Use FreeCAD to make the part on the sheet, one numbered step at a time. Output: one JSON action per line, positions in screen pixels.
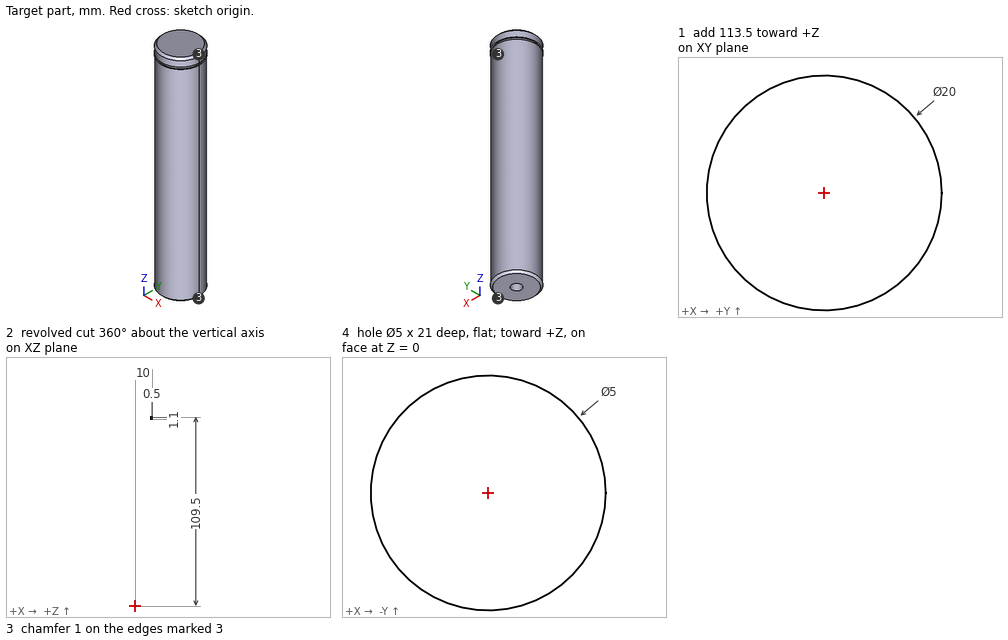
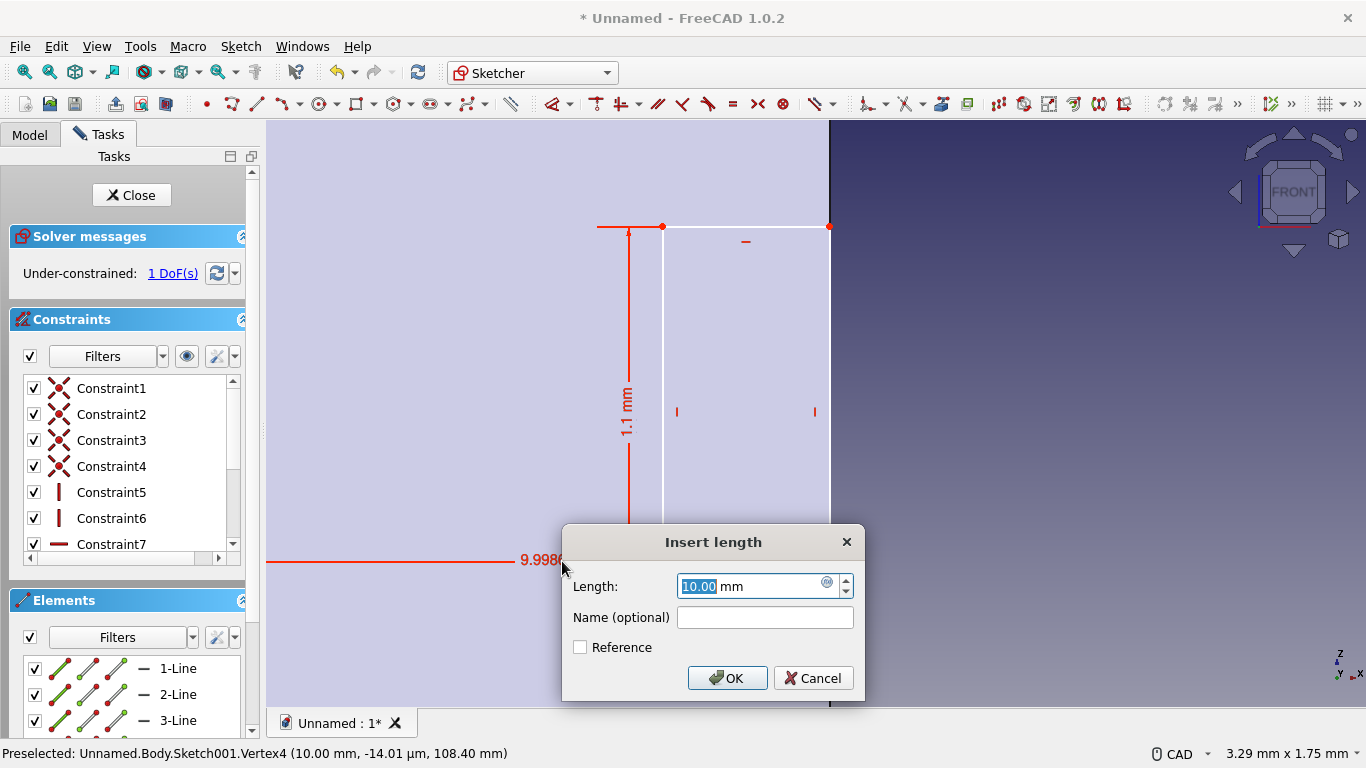
{"action": "type", "text": "10"}
{"action": "key", "text": "Return"}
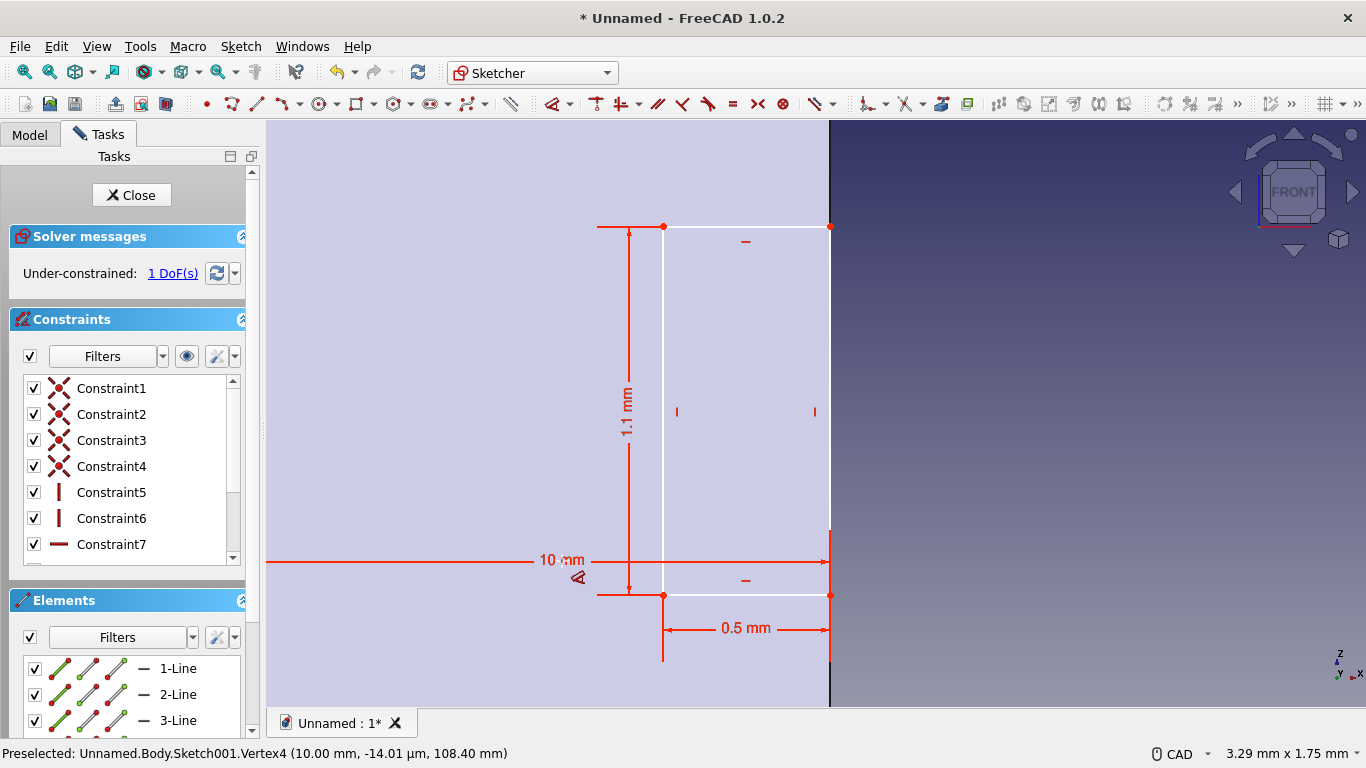
{"action": "left_click", "coordinate": [663, 227]}
{"action": "left_click", "coordinate": [697, 453]}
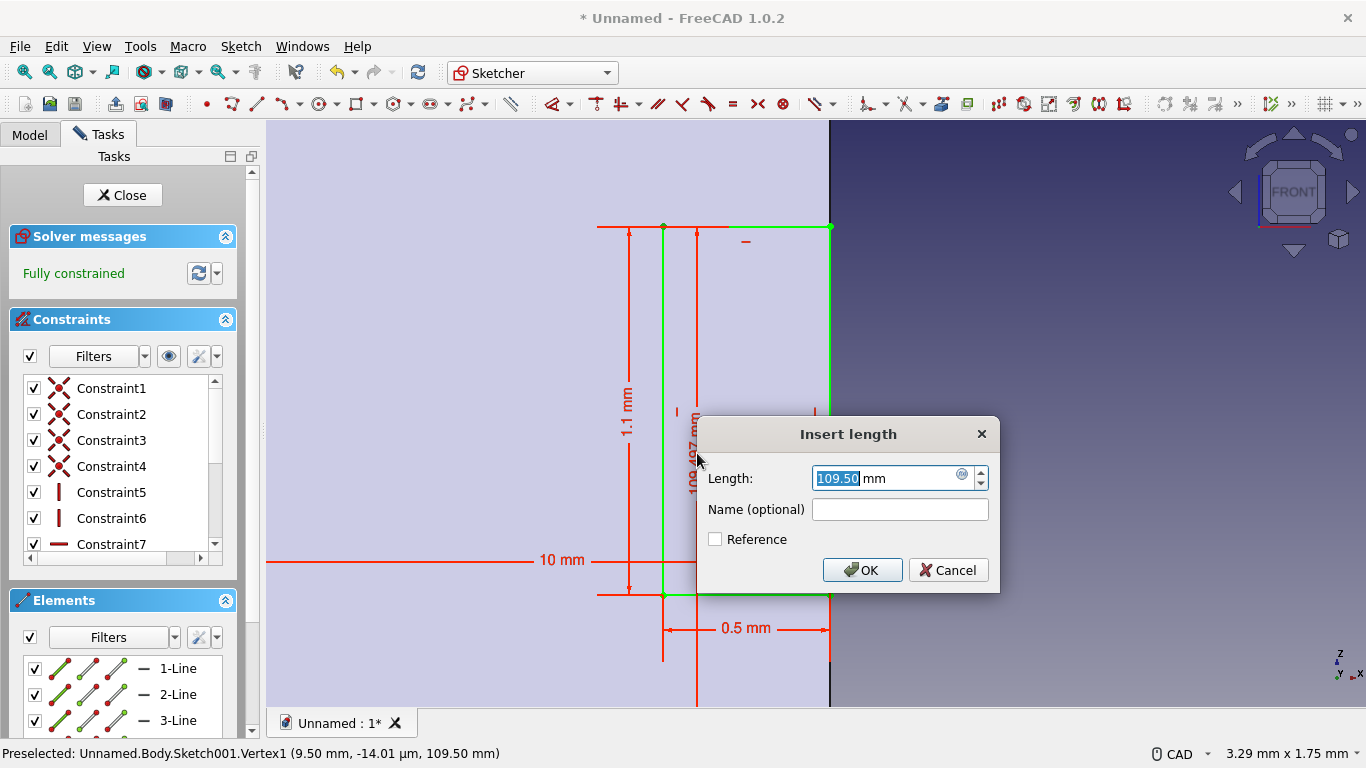
{"action": "type", "text": "109.5"}
{"action": "key", "text": "Return"}
{"action": "key", "text": "Escape"}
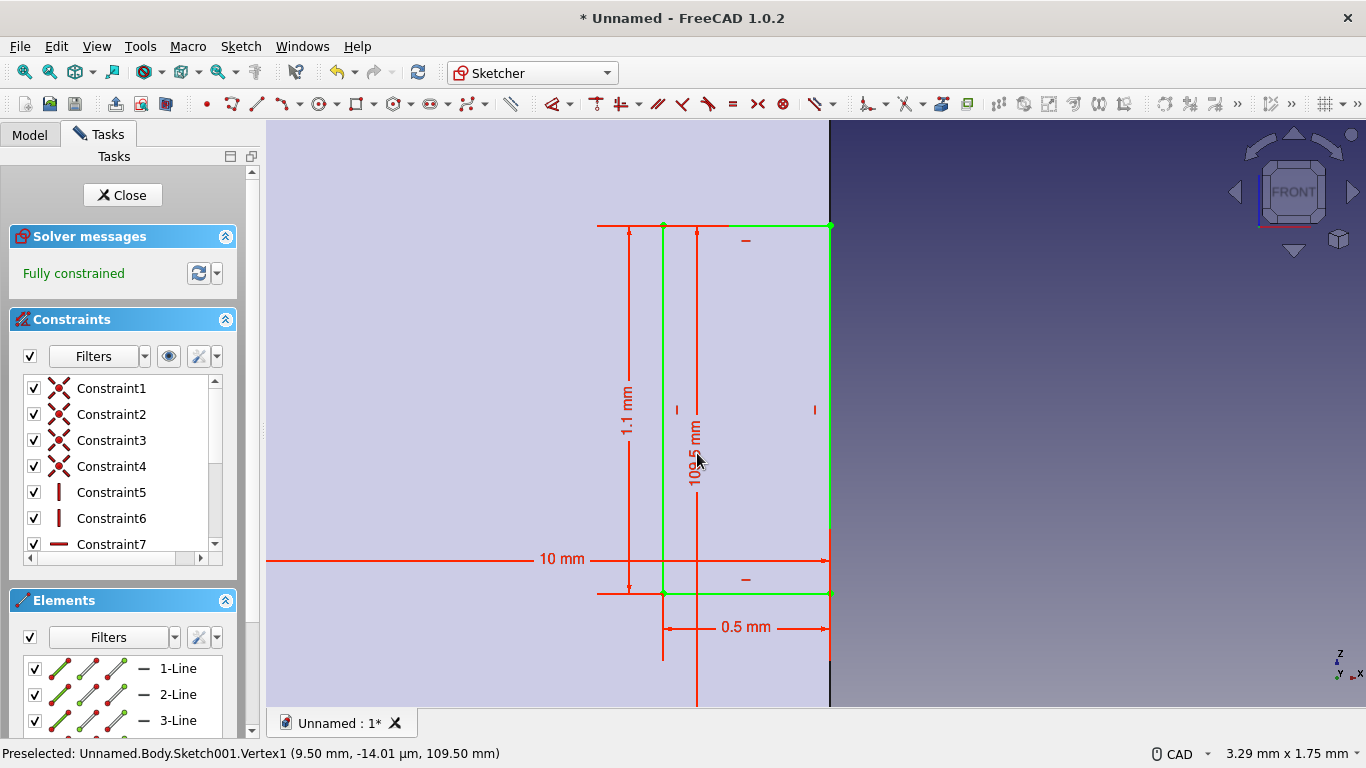
{"action": "left_click", "coordinate": [123, 195]}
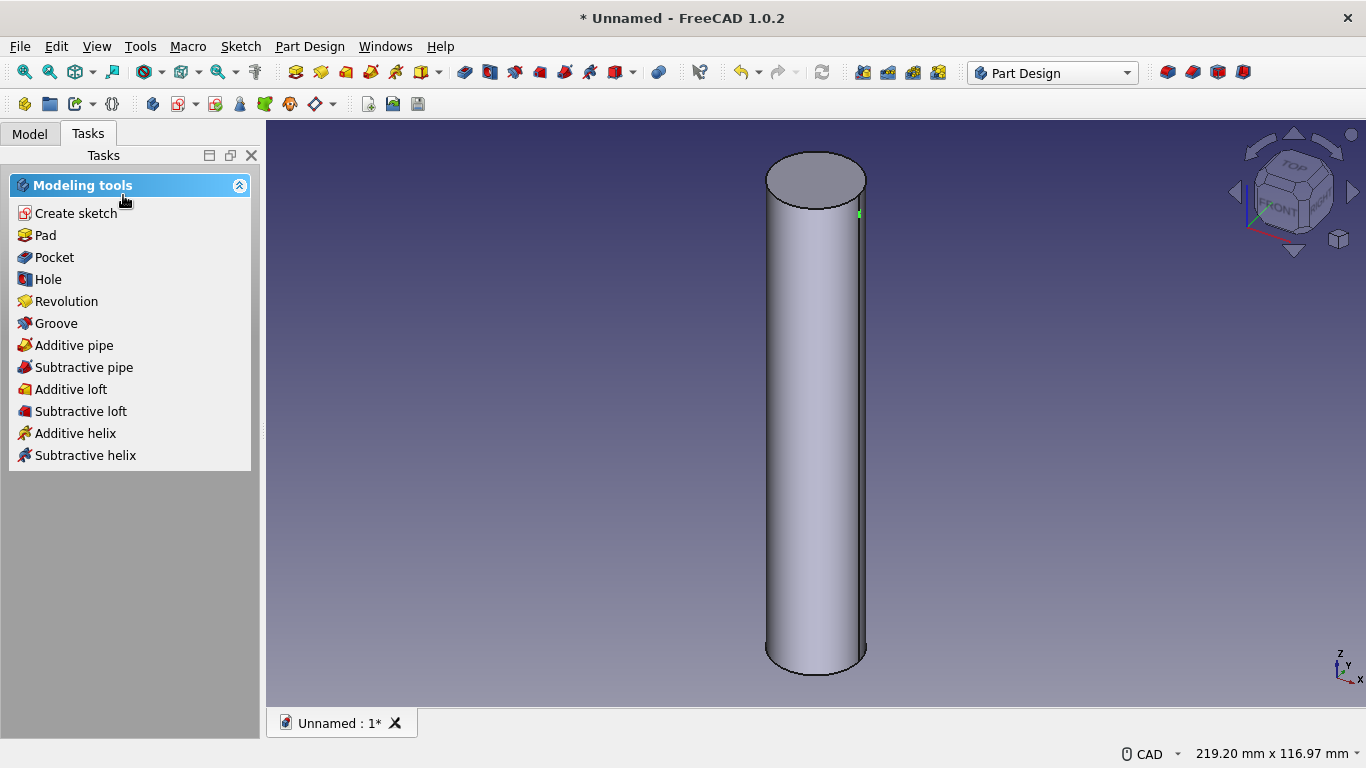
{"action": "left_click", "coordinate": [515, 72]}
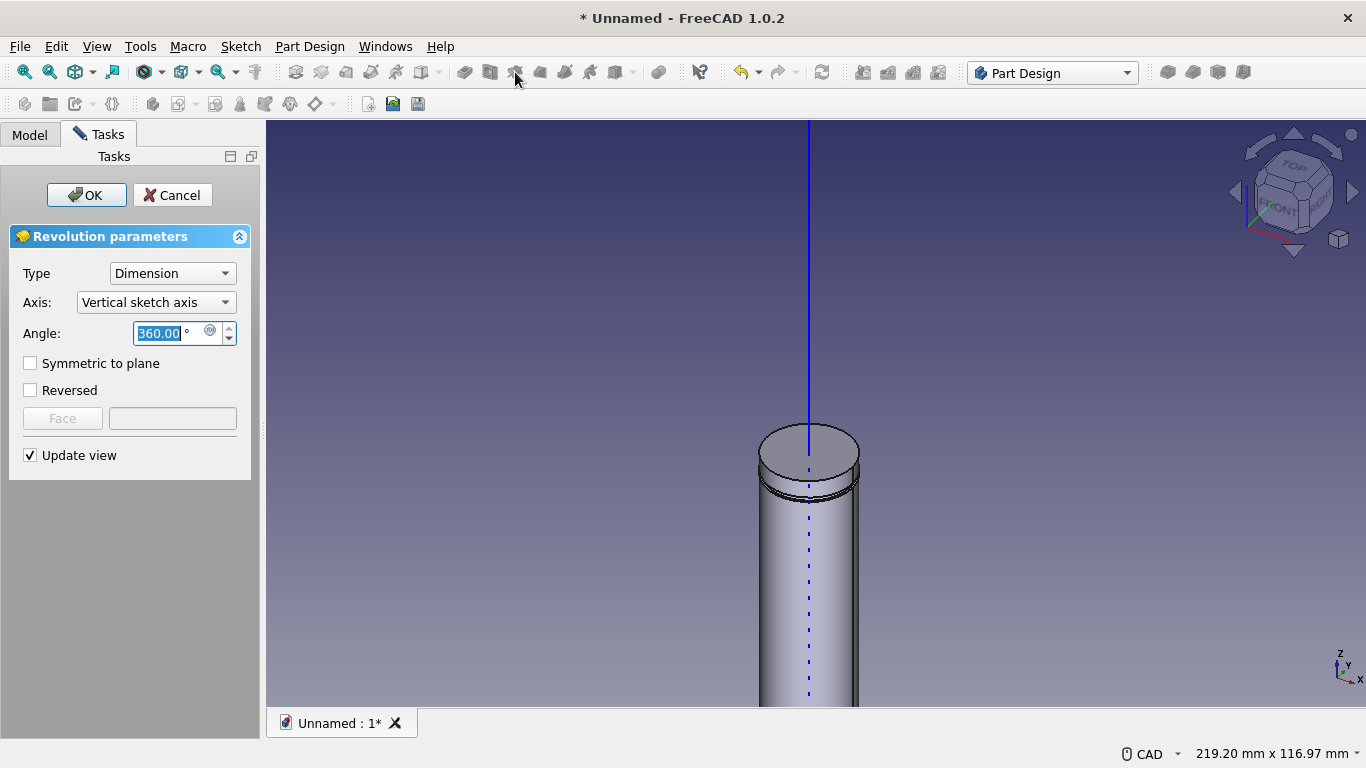
{"action": "left_click", "coordinate": [87, 195]}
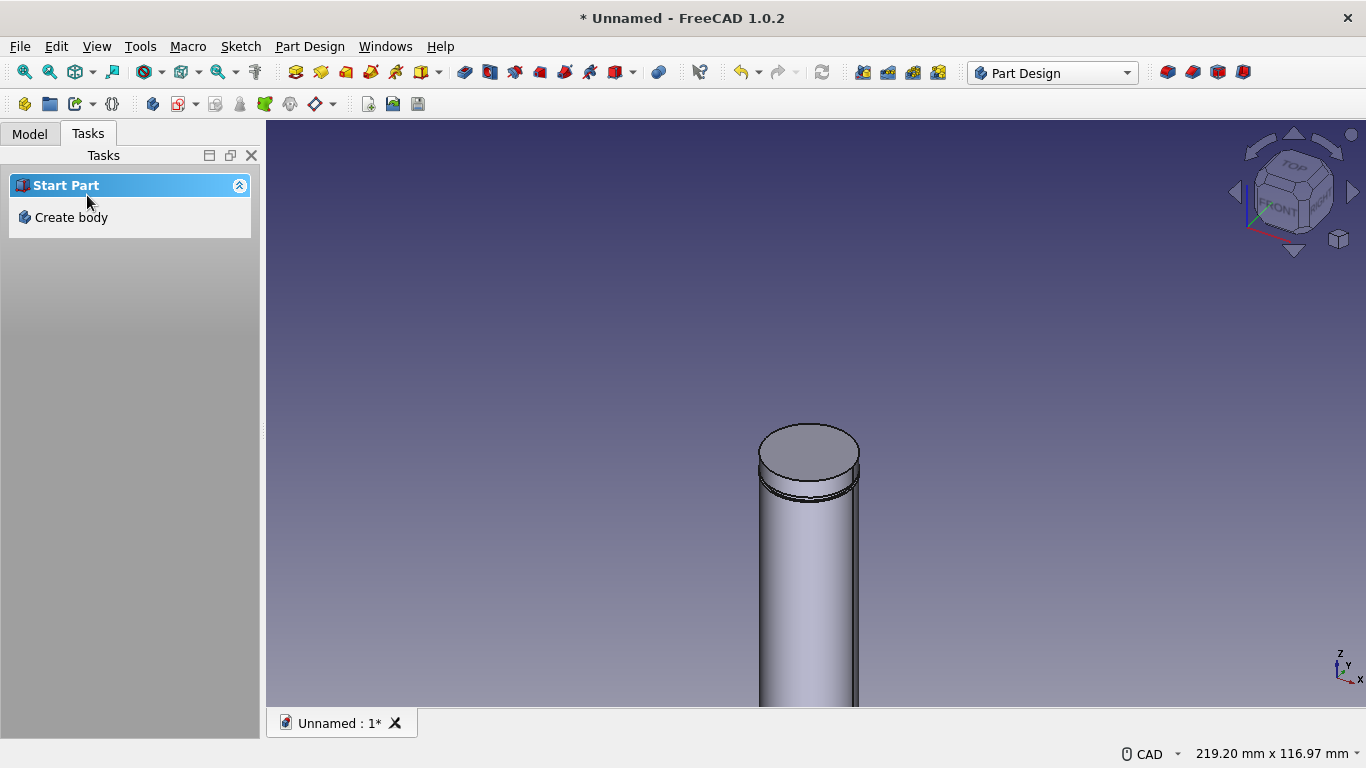
{"action": "key", "text": "v f"}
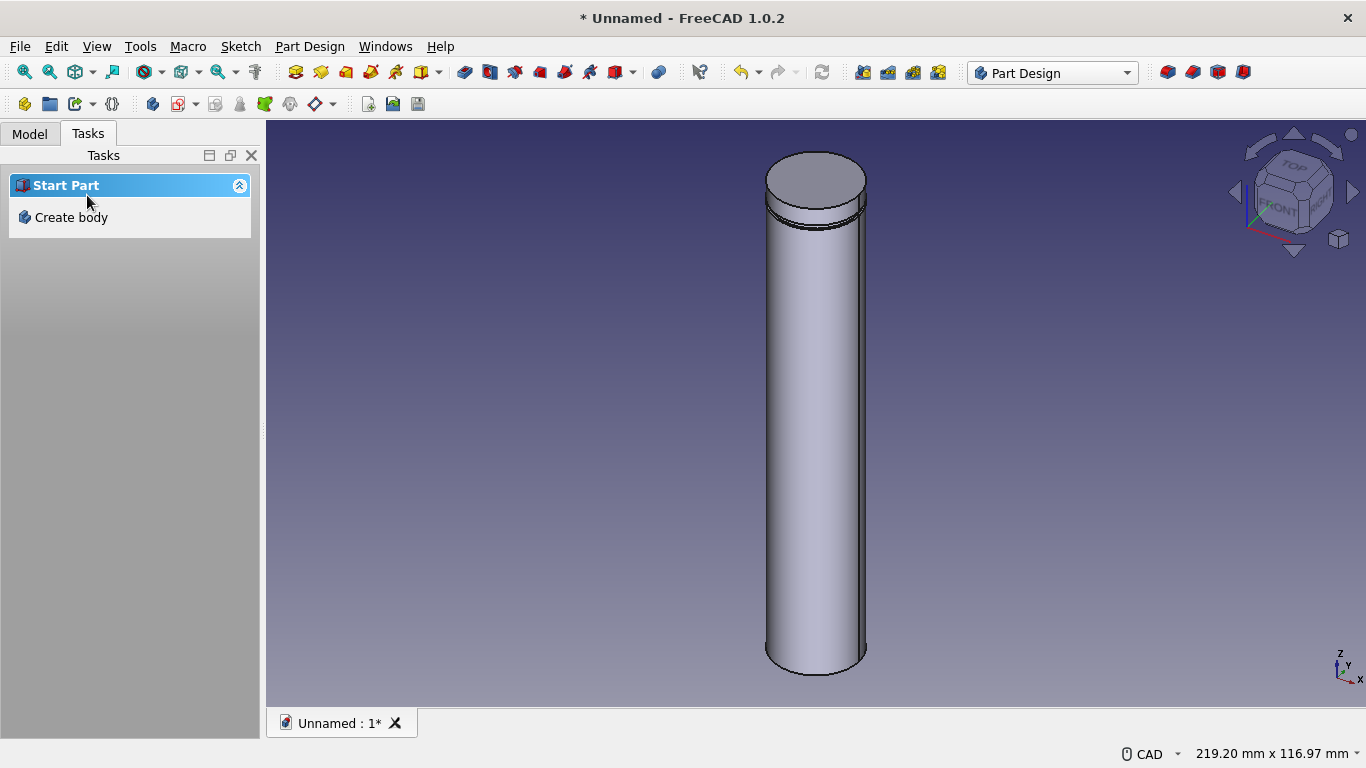
{"action": "left_click", "coordinate": [766, 182]}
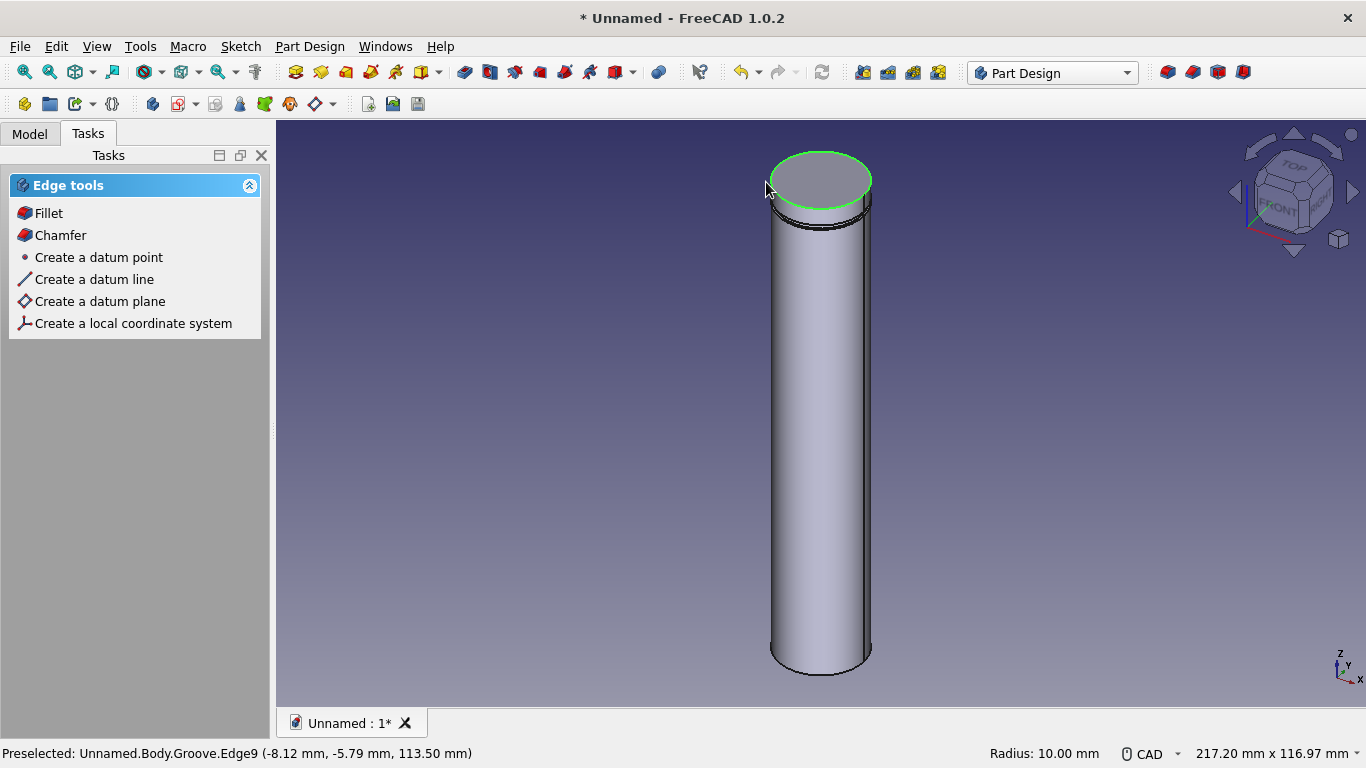
{"action": "key", "text": "0"}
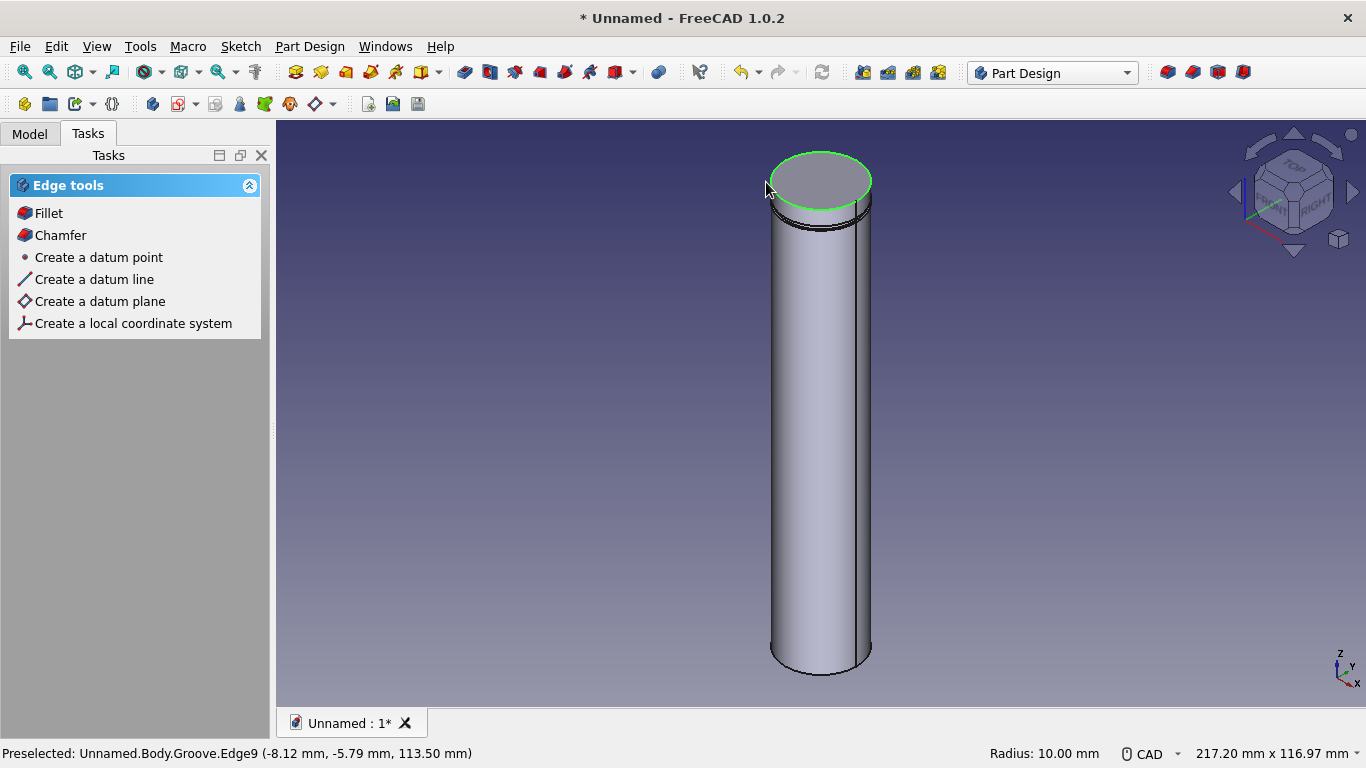
{"action": "key", "text": "2"}